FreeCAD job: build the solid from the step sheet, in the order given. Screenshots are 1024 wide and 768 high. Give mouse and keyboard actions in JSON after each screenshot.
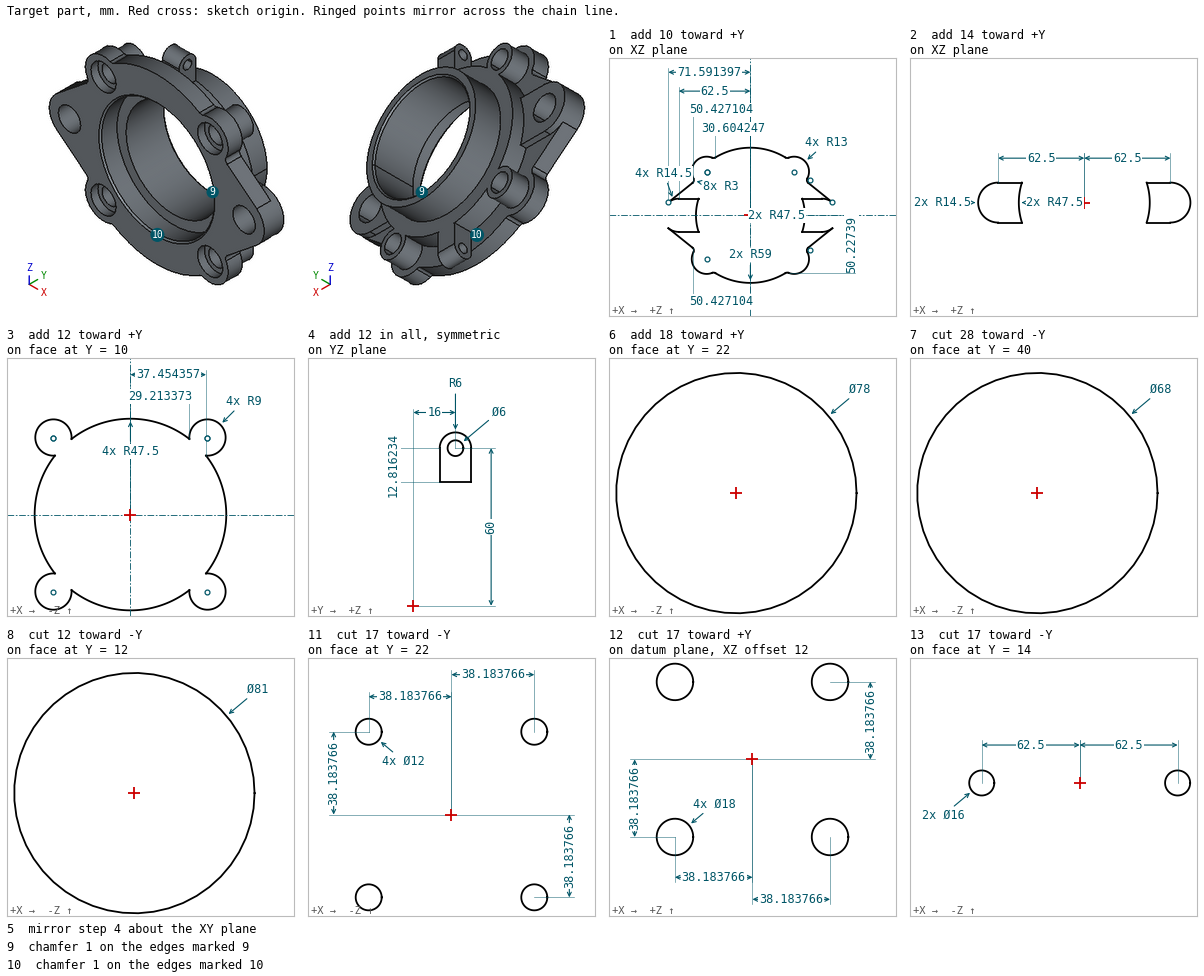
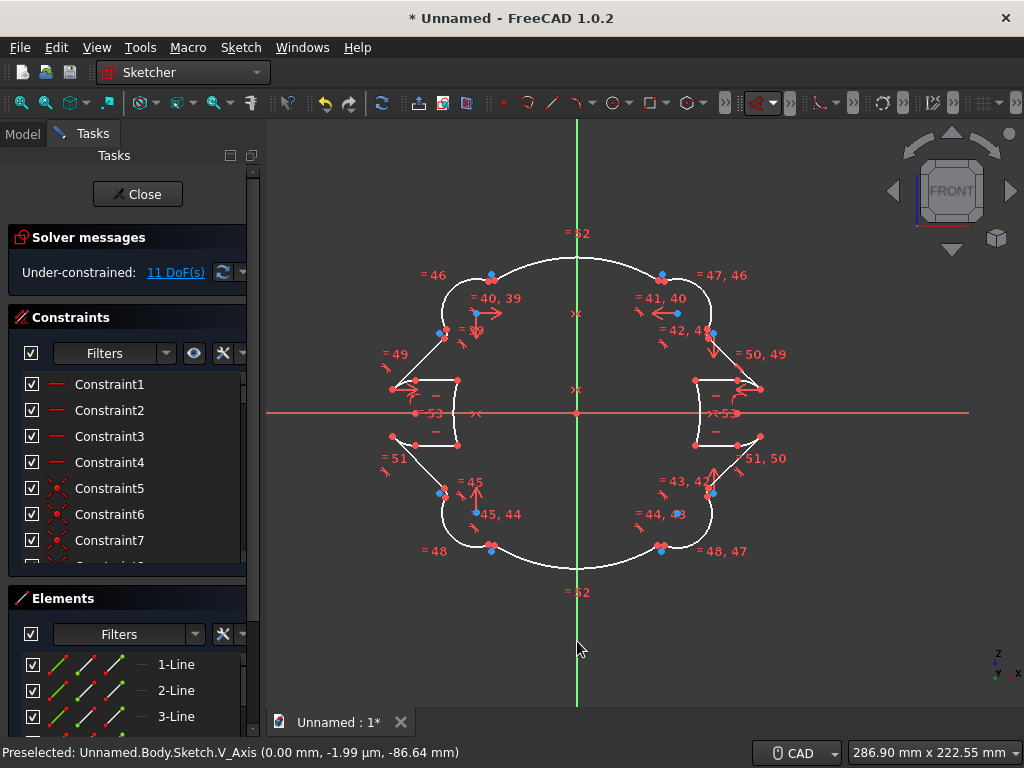
{"action": "scroll", "coordinate": [411, 381], "scroll_direction": "up", "scroll_amount": 5}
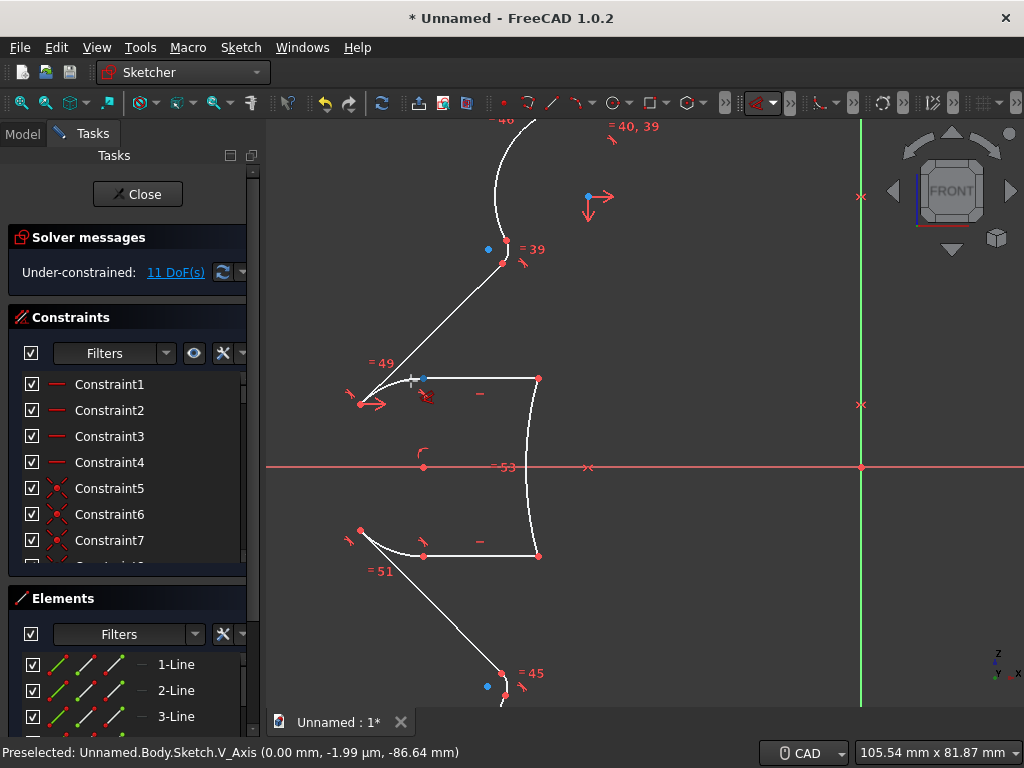
{"action": "left_click", "coordinate": [409, 380]}
{"action": "left_click", "coordinate": [463, 354]}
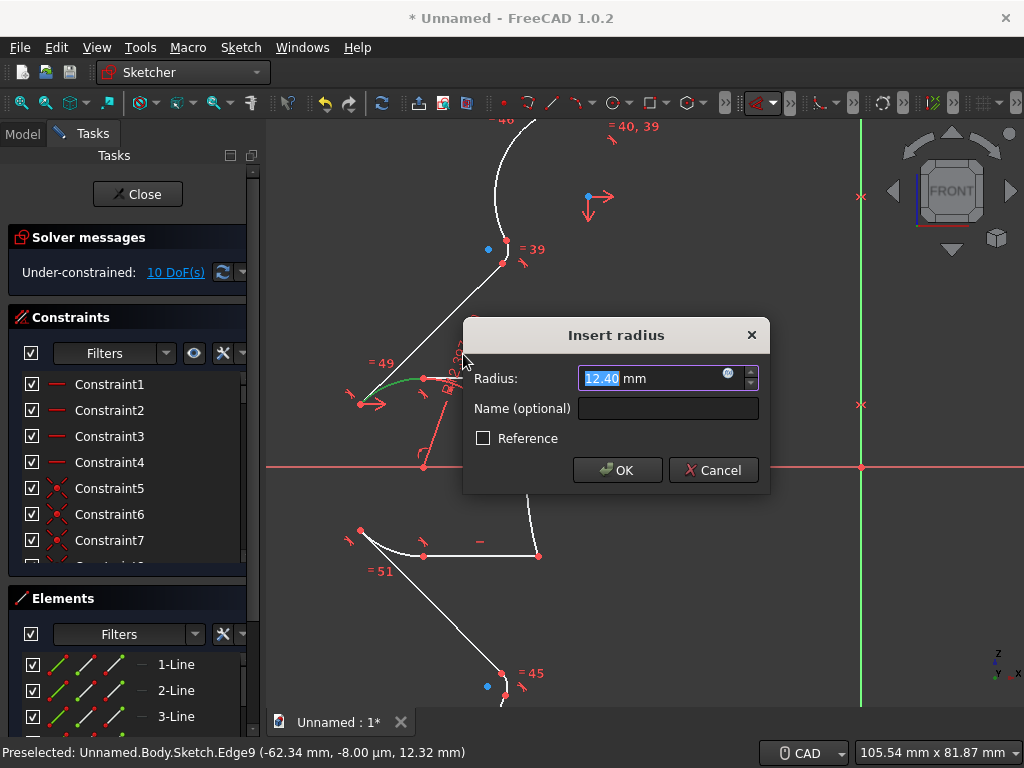
{"action": "type", "text": "14.5"}
{"action": "key", "text": "Return"}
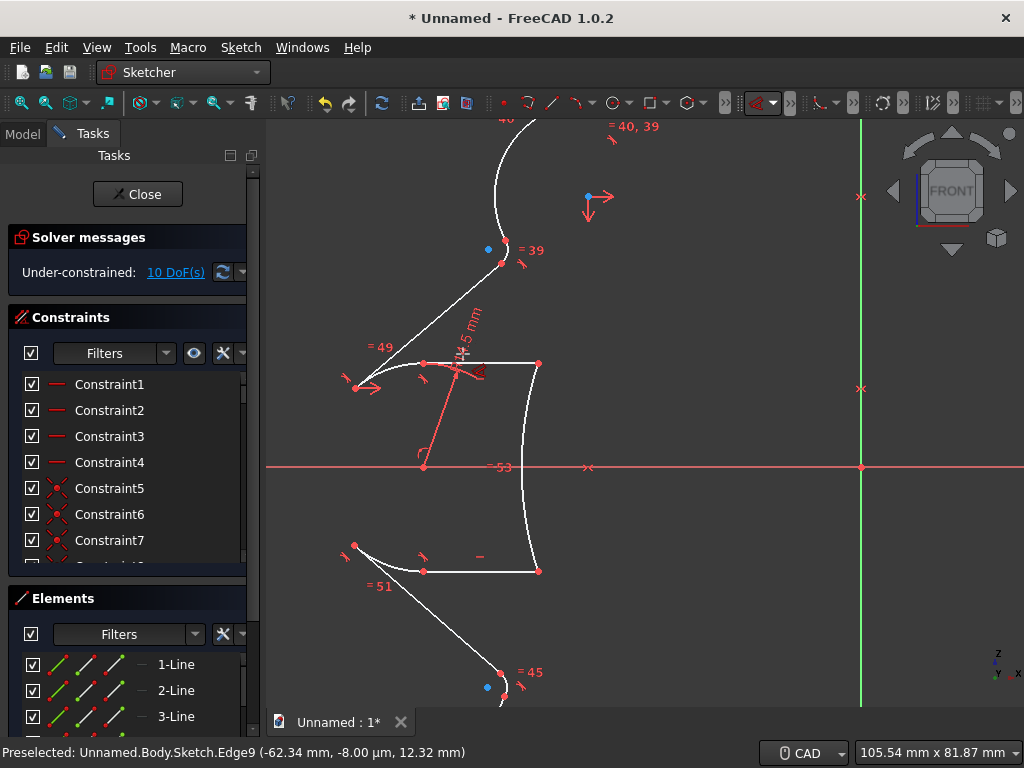
{"action": "scroll", "coordinate": [508, 253], "scroll_direction": "up", "scroll_amount": 4}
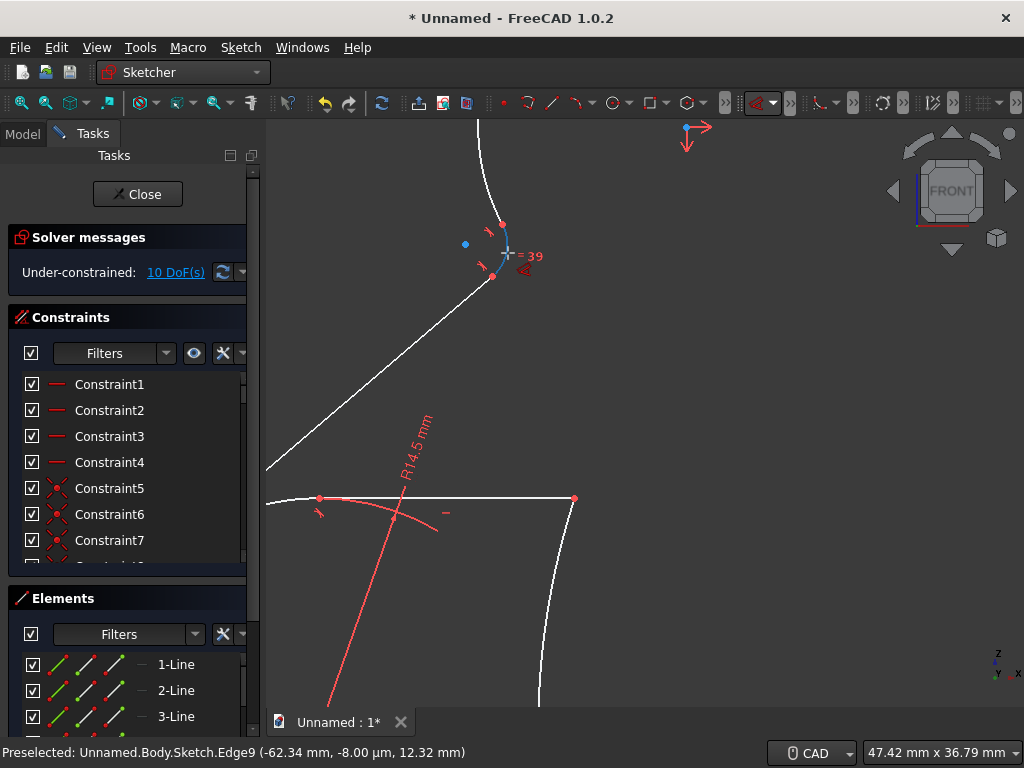
{"action": "left_click", "coordinate": [507, 252]}
{"action": "left_click", "coordinate": [538, 258]}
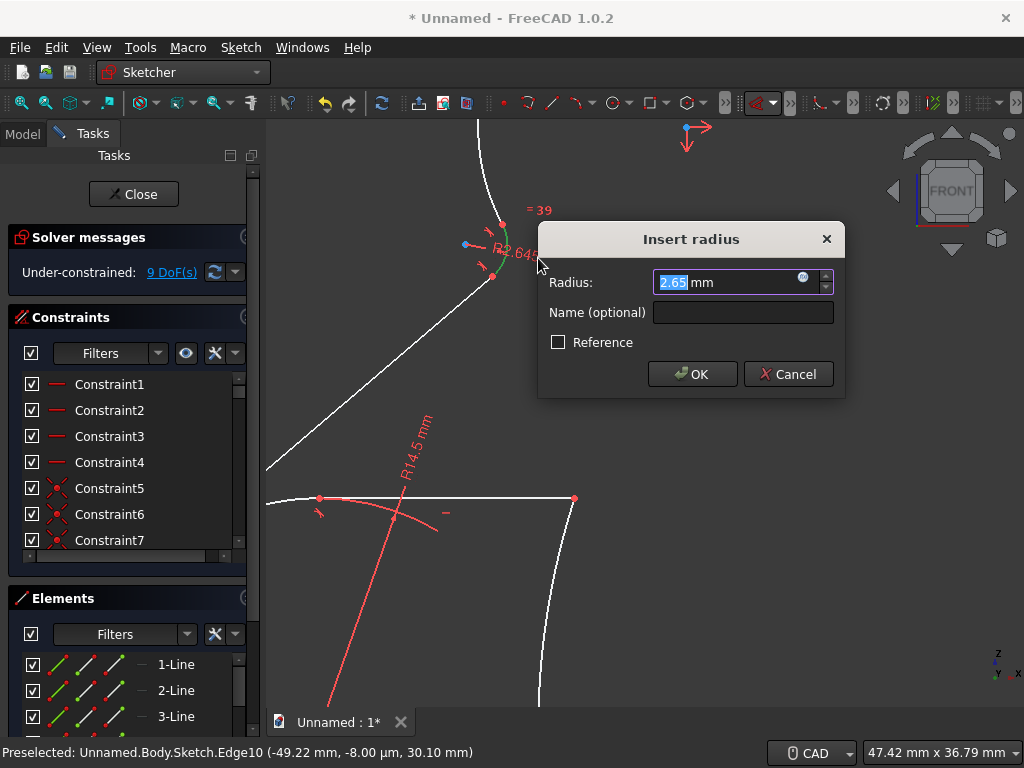
{"action": "type", "text": "3"}
{"action": "key", "text": "Return"}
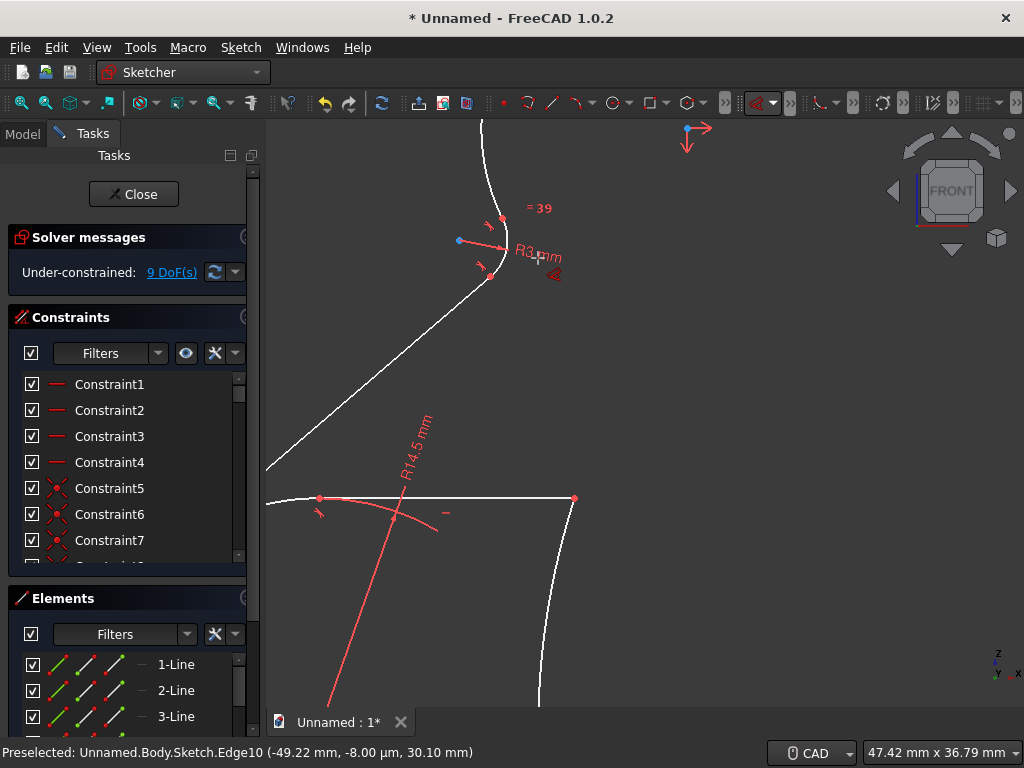
{"action": "scroll", "coordinate": [434, 350], "scroll_direction": "down", "scroll_amount": 9}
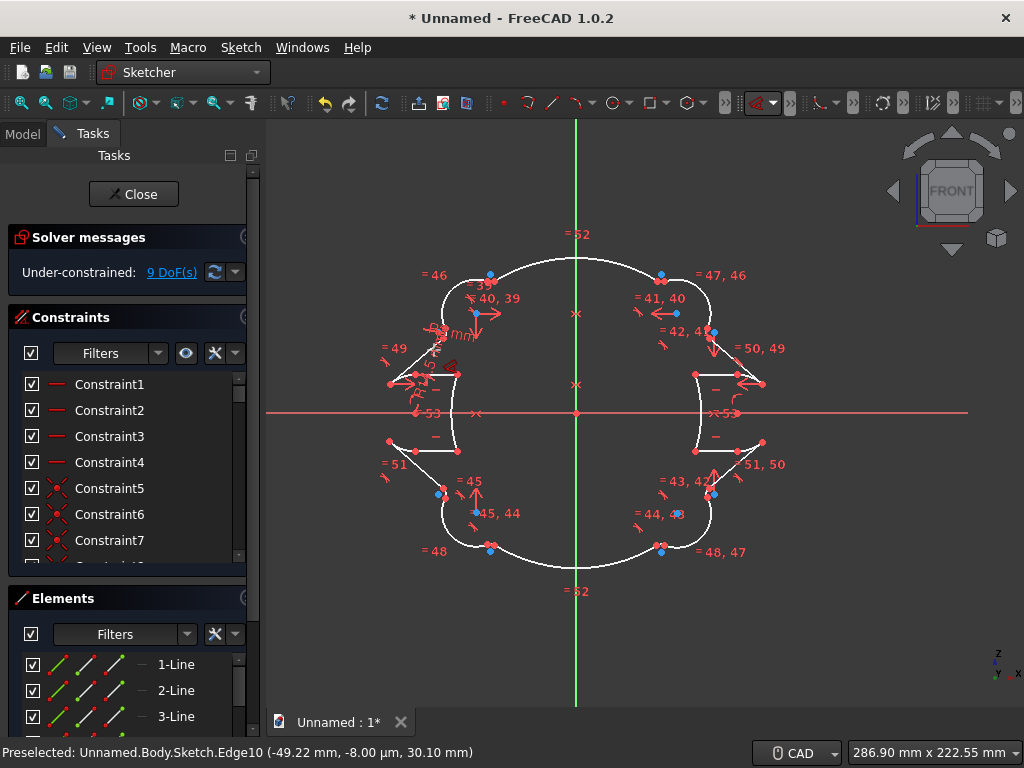
{"action": "left_click", "coordinate": [464, 282]}
{"action": "left_click", "coordinate": [453, 252]}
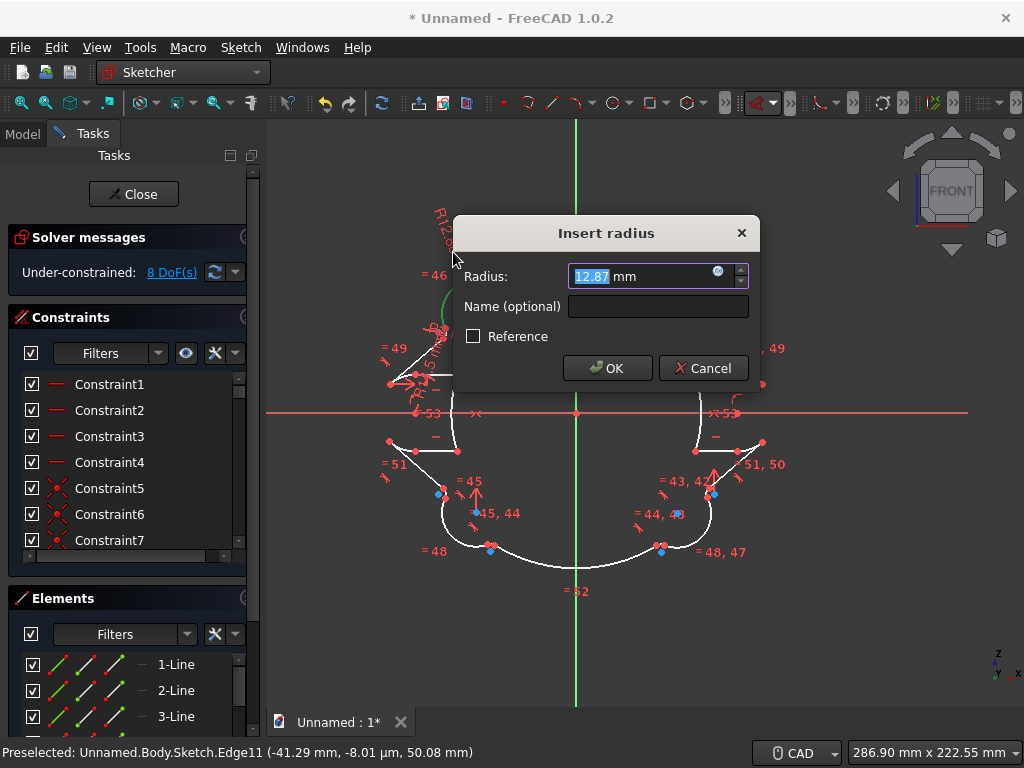
{"action": "type", "text": "13"}
{"action": "key", "text": "Return"}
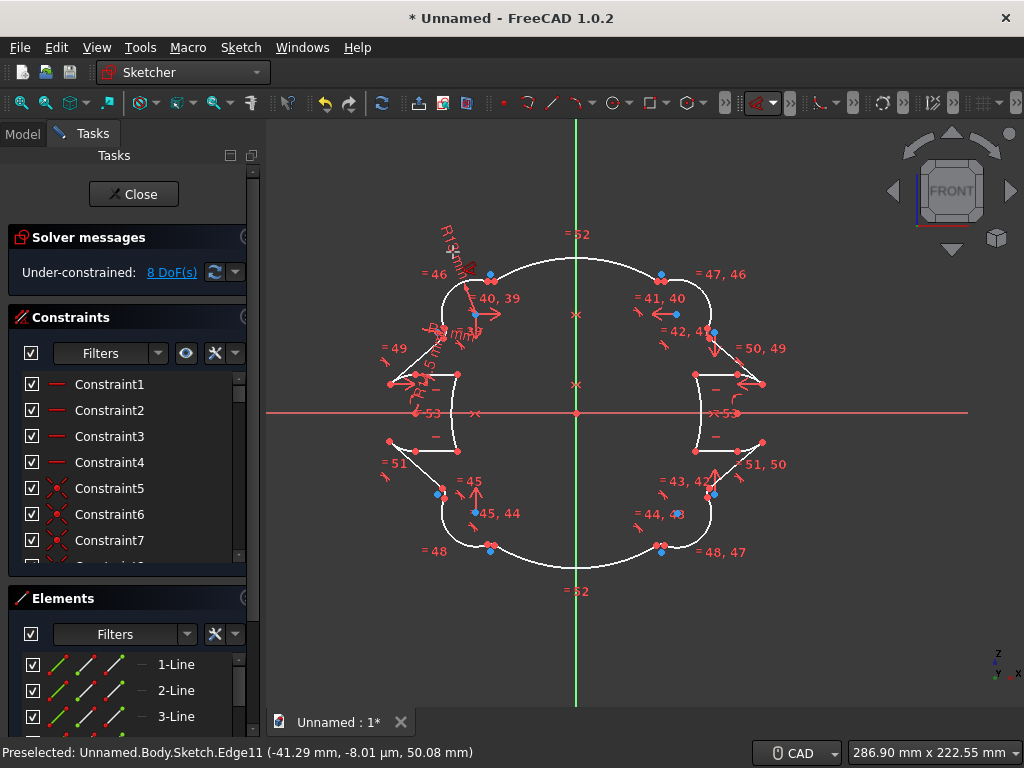
{"action": "left_click", "coordinate": [610, 262]}
{"action": "left_click", "coordinate": [617, 231]}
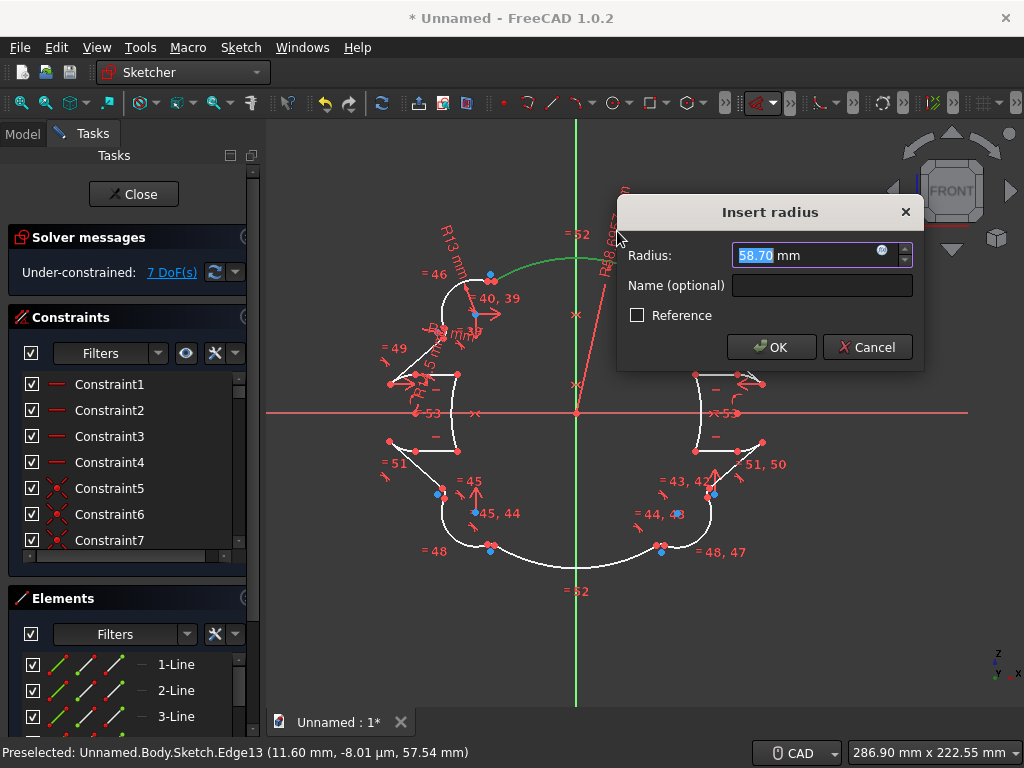
{"action": "type", "text": "59"}
{"action": "key", "text": "Return"}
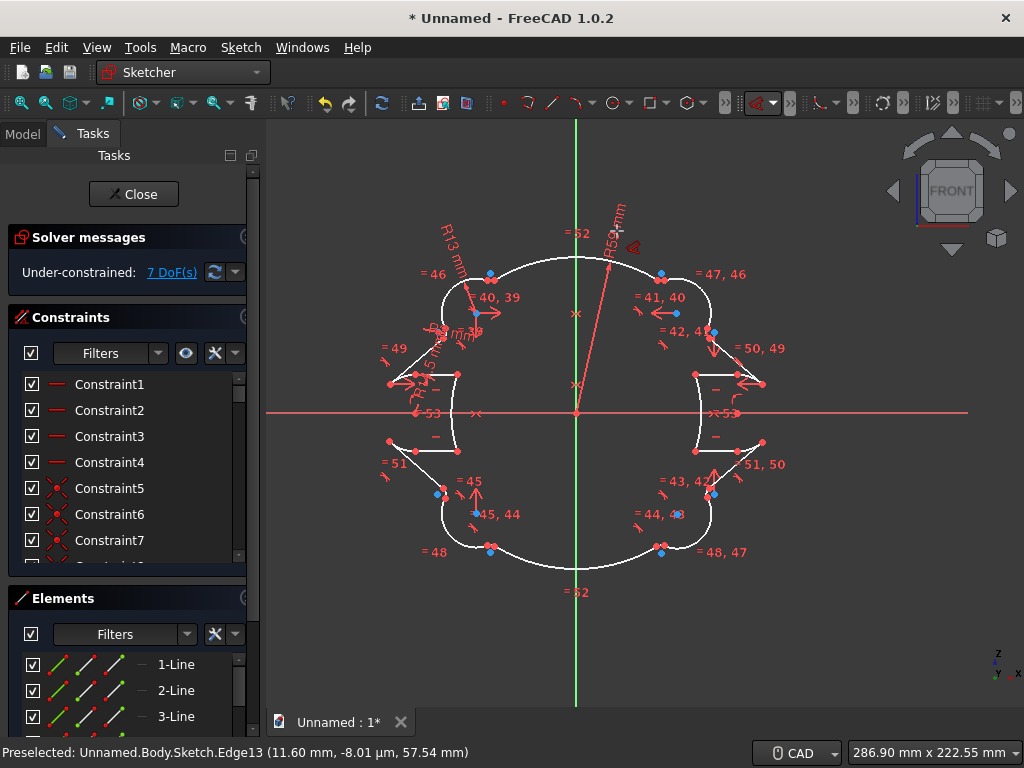
{"action": "left_click", "coordinate": [700, 429]}
{"action": "left_click", "coordinate": [732, 433]}